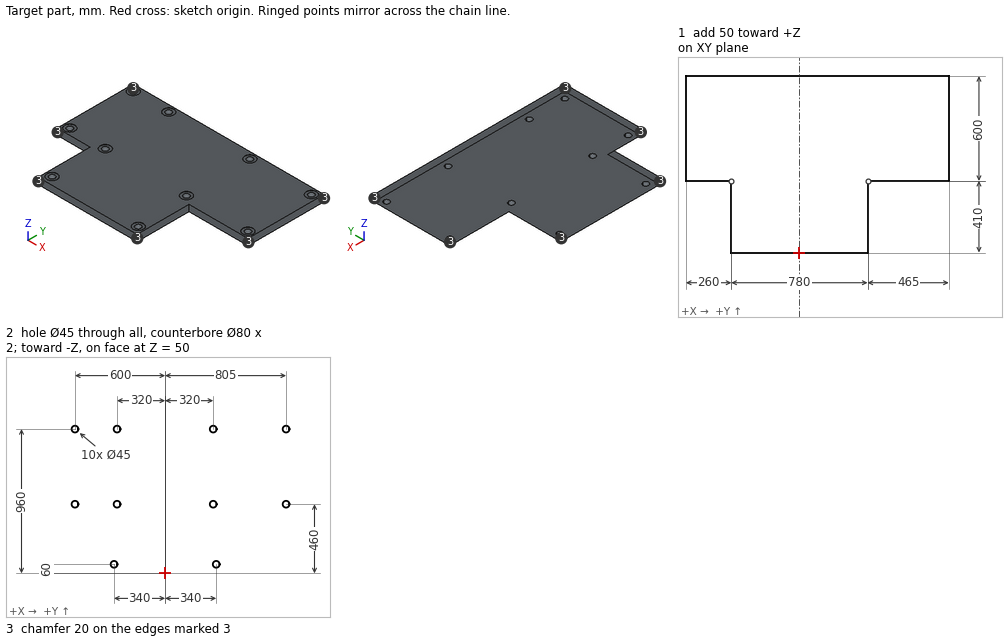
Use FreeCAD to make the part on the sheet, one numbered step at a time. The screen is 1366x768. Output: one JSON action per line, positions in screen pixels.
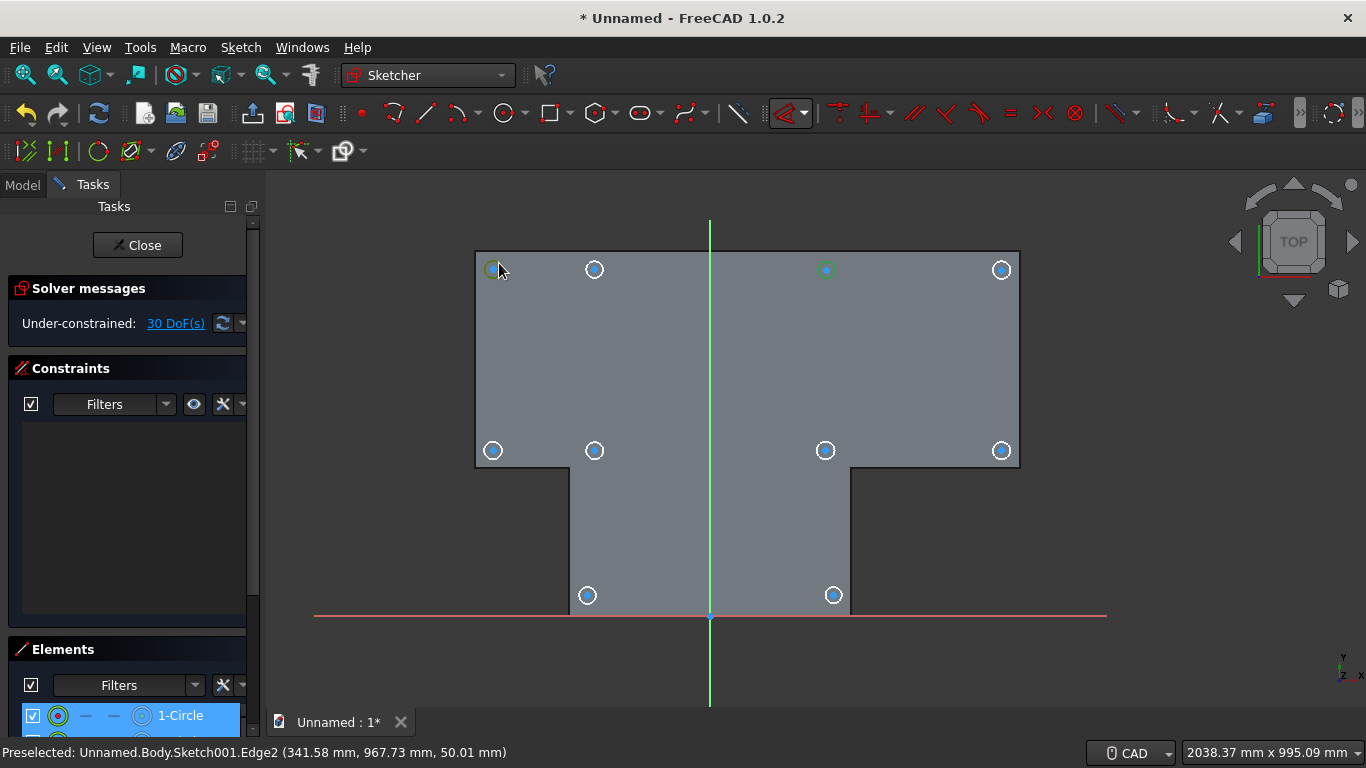
{"action": "scroll", "coordinate": [1008, 264], "scroll_direction": "up", "scroll_amount": 3}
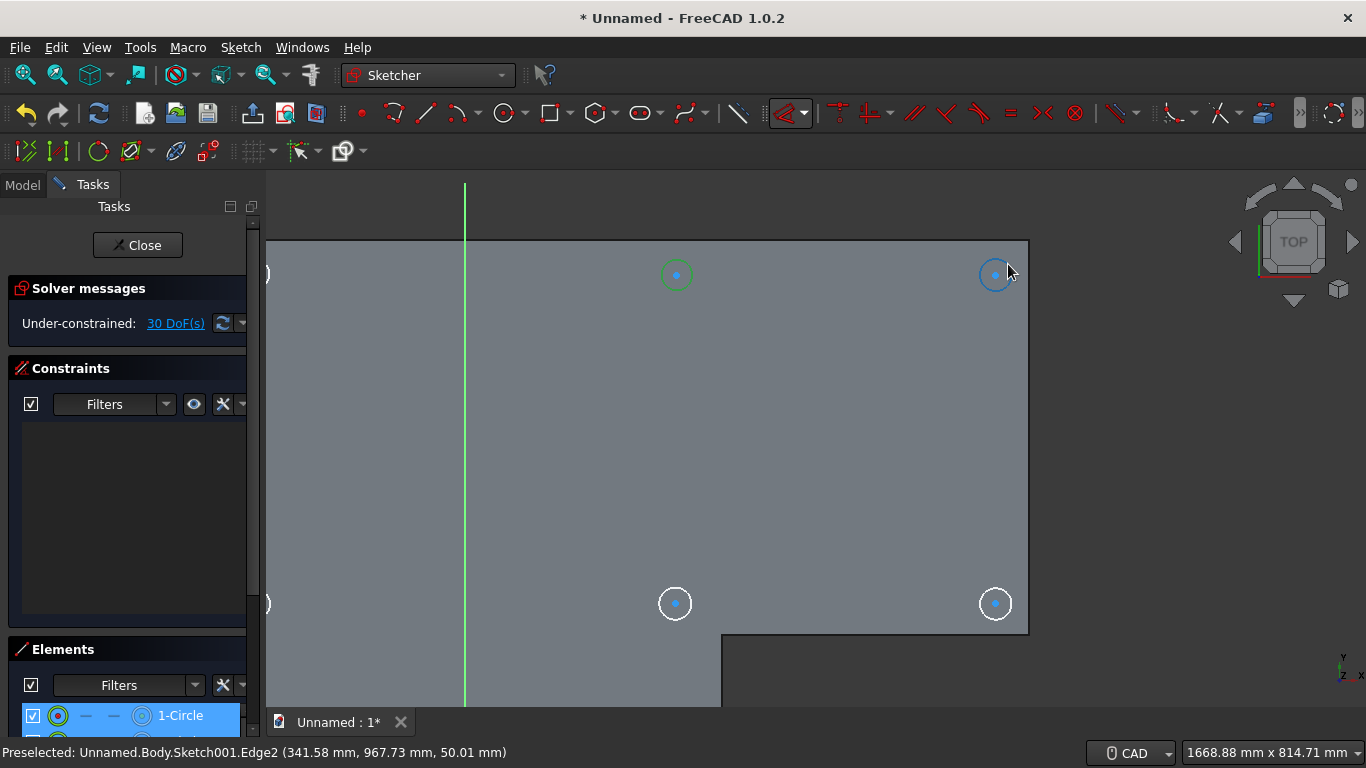
{"action": "left_click", "coordinate": [1007, 264]}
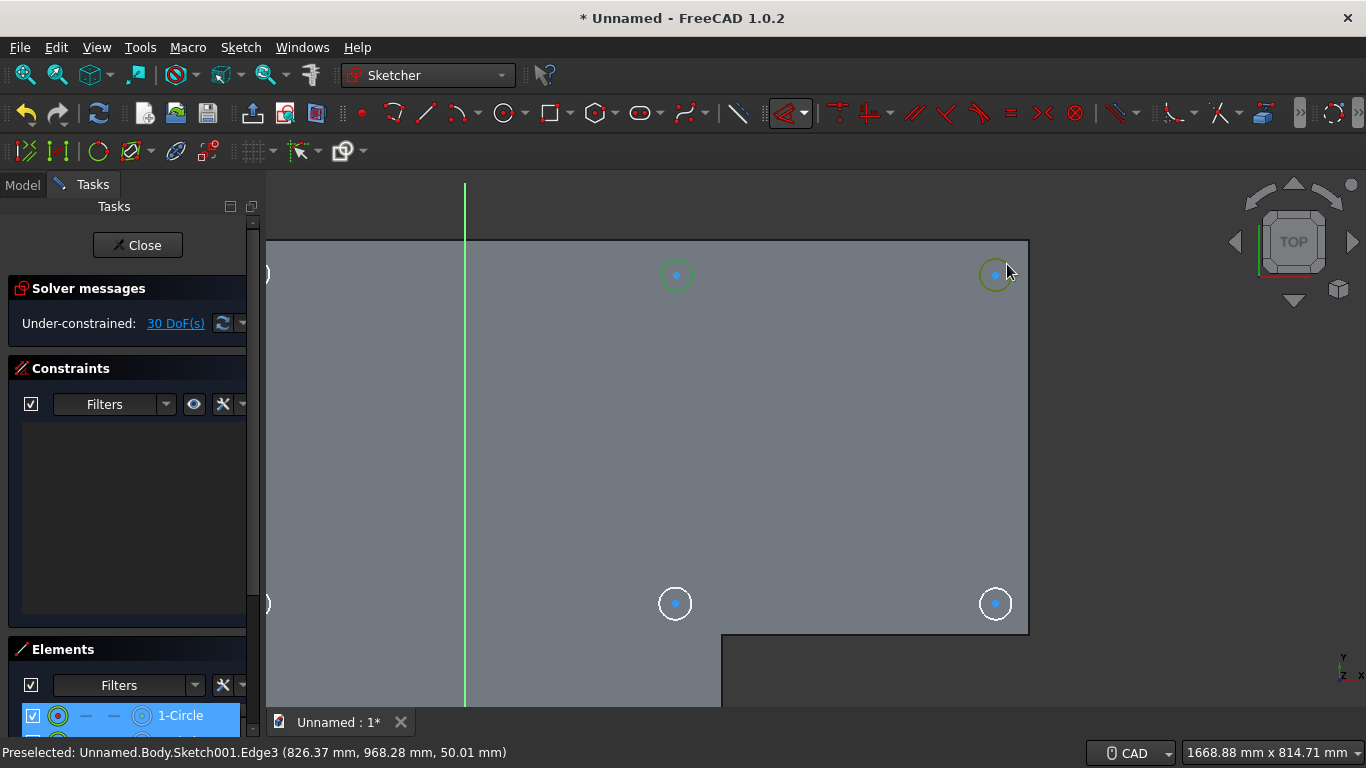
{"action": "scroll", "coordinate": [1009, 264], "scroll_direction": "down", "scroll_amount": 3}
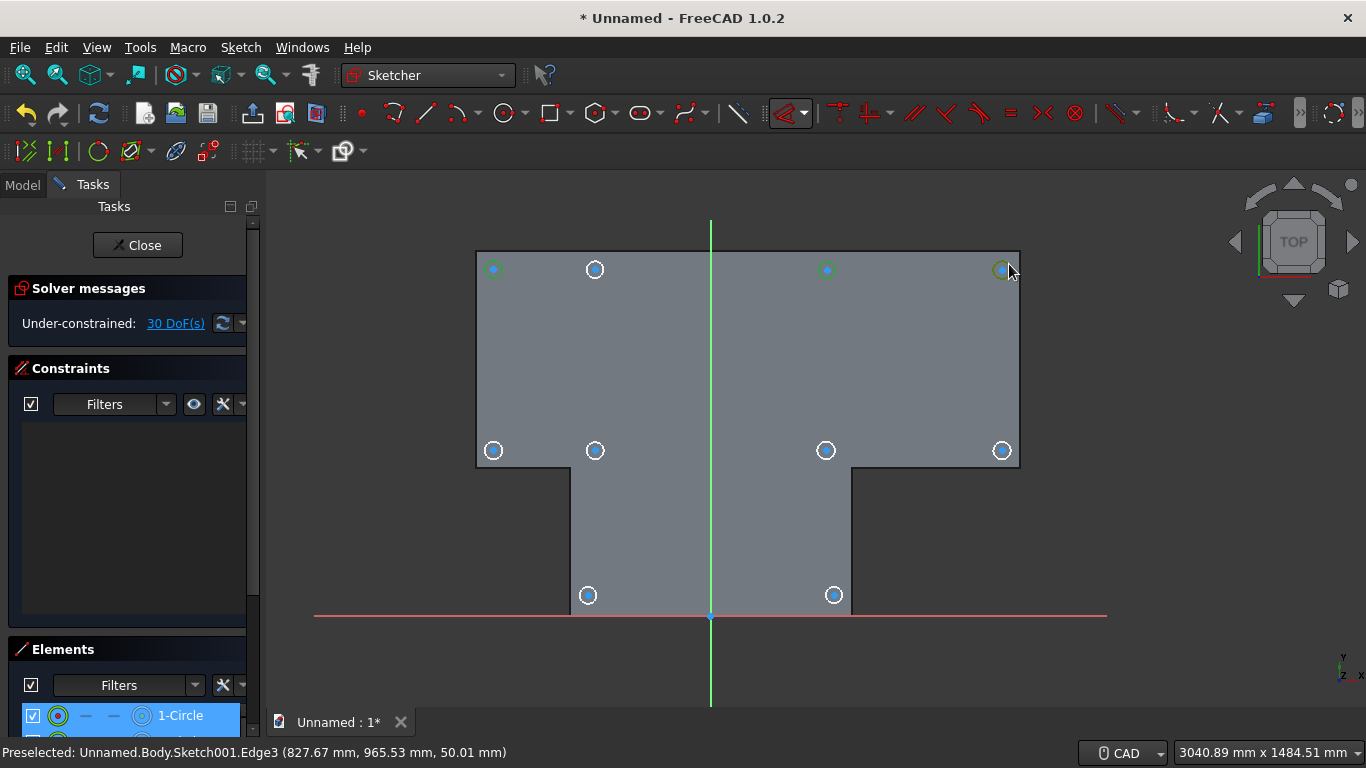
{"action": "scroll", "coordinate": [594, 589], "scroll_direction": "up", "scroll_amount": 3}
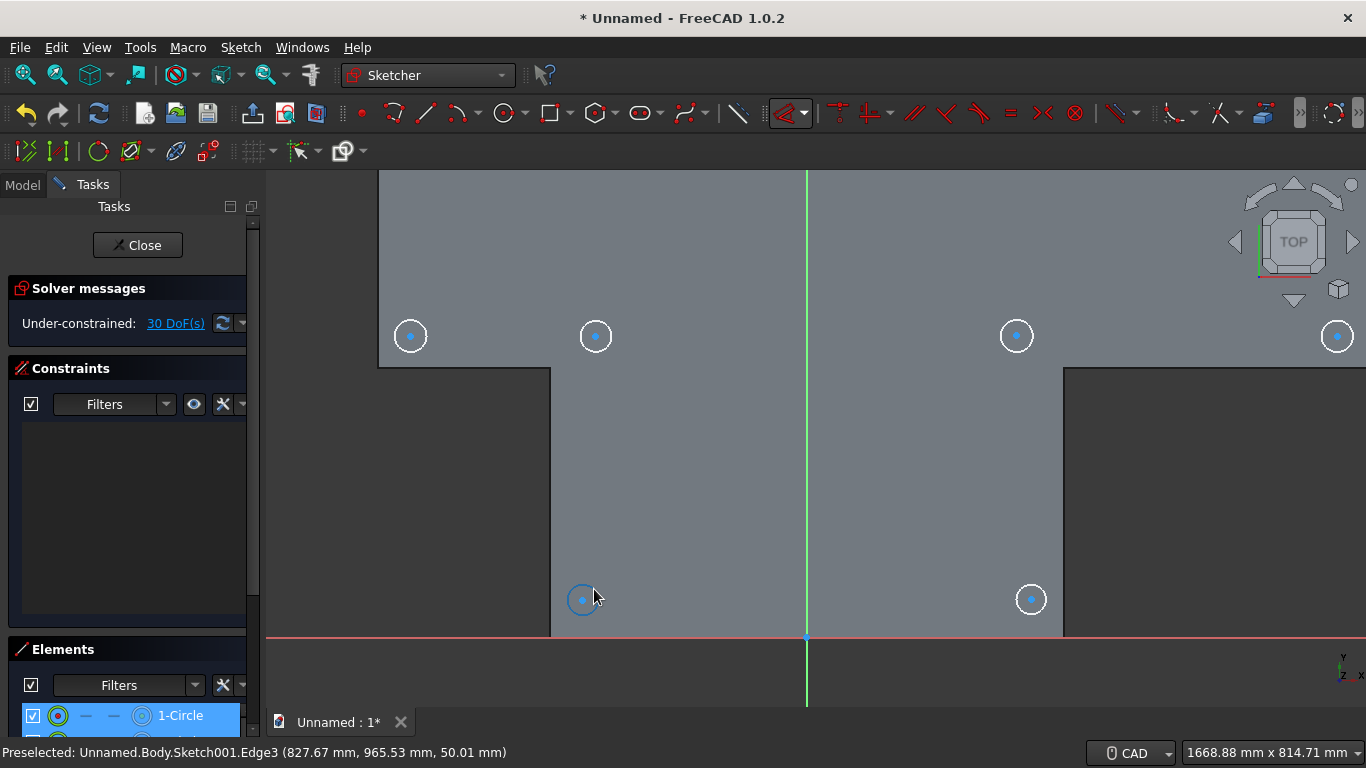
{"action": "left_click", "coordinate": [594, 589]}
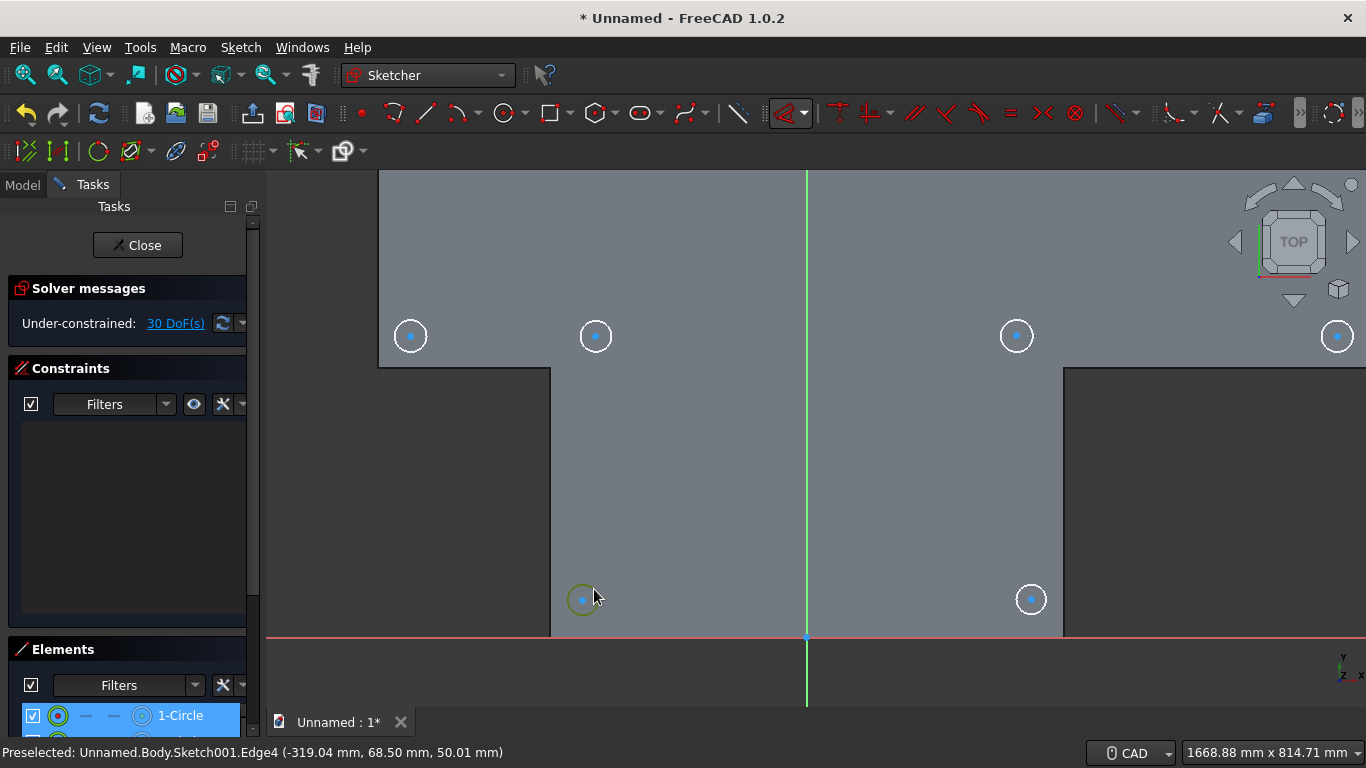
{"action": "left_click", "coordinate": [1042, 589]}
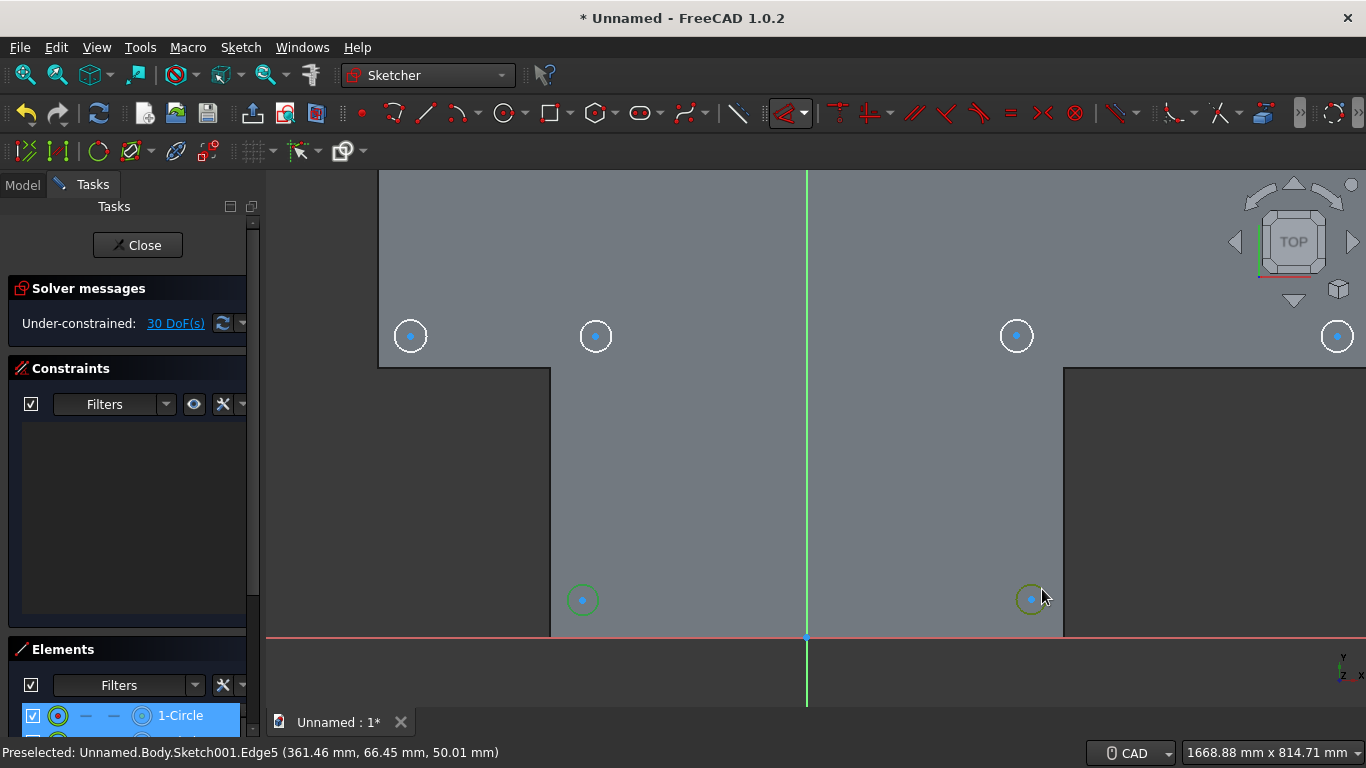
{"action": "scroll", "coordinate": [593, 590], "scroll_direction": "down", "scroll_amount": 3}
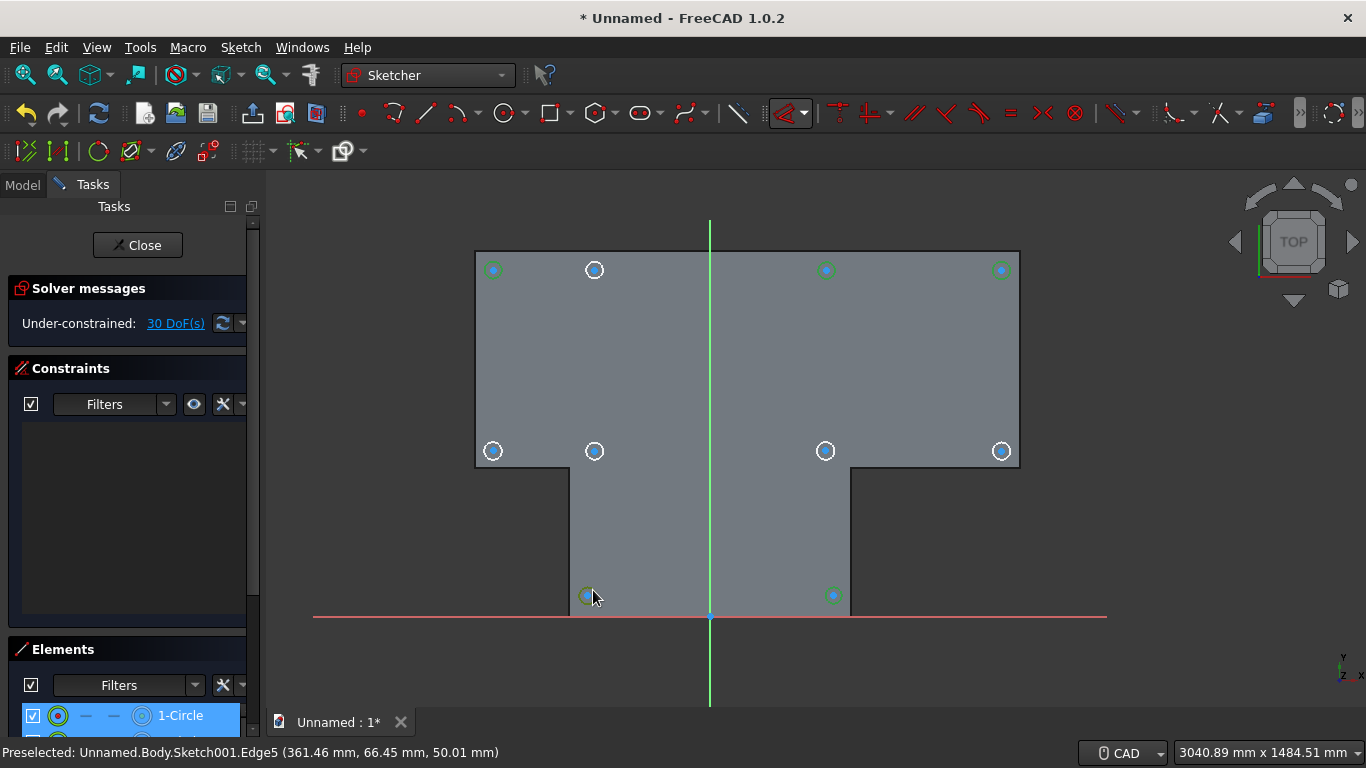
{"action": "scroll", "coordinate": [600, 264], "scroll_direction": "up", "scroll_amount": 3}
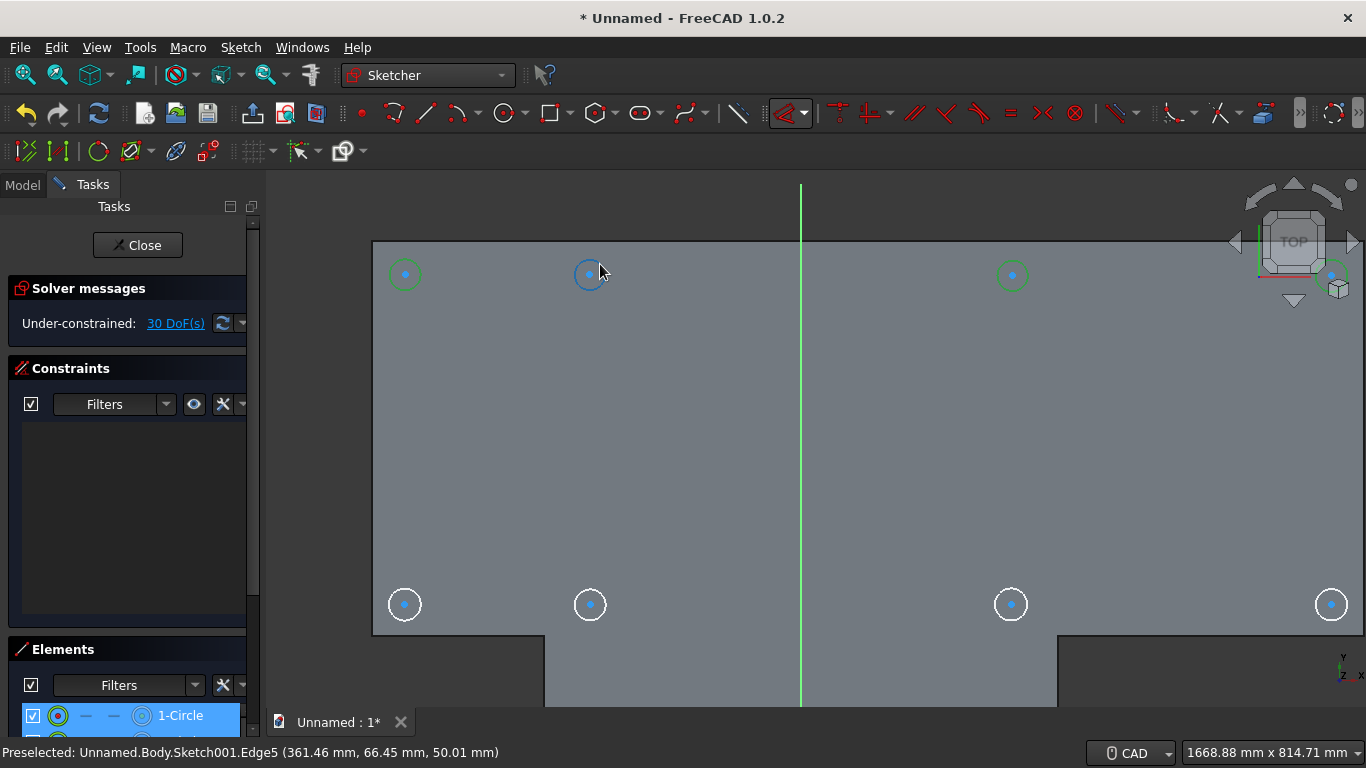
{"action": "left_click", "coordinate": [601, 264]}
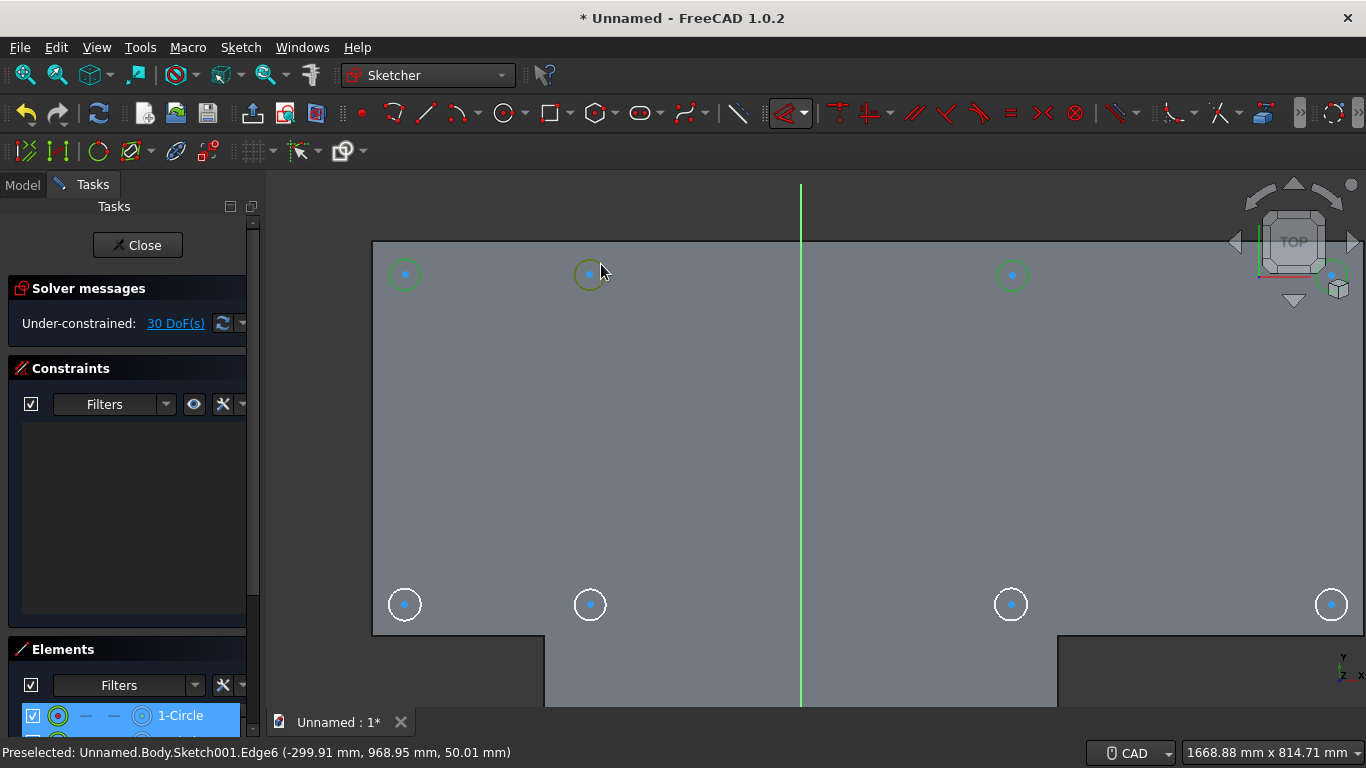
{"action": "scroll", "coordinate": [600, 263], "scroll_direction": "down", "scroll_amount": 3}